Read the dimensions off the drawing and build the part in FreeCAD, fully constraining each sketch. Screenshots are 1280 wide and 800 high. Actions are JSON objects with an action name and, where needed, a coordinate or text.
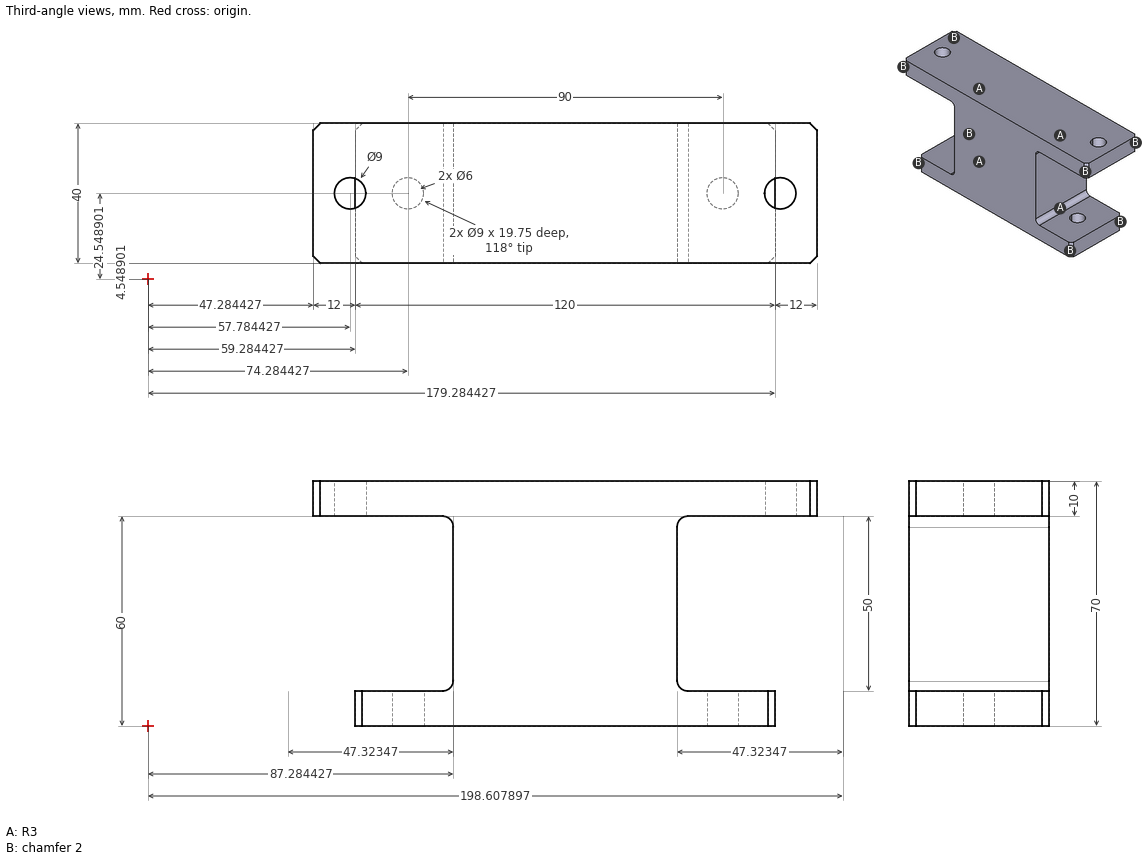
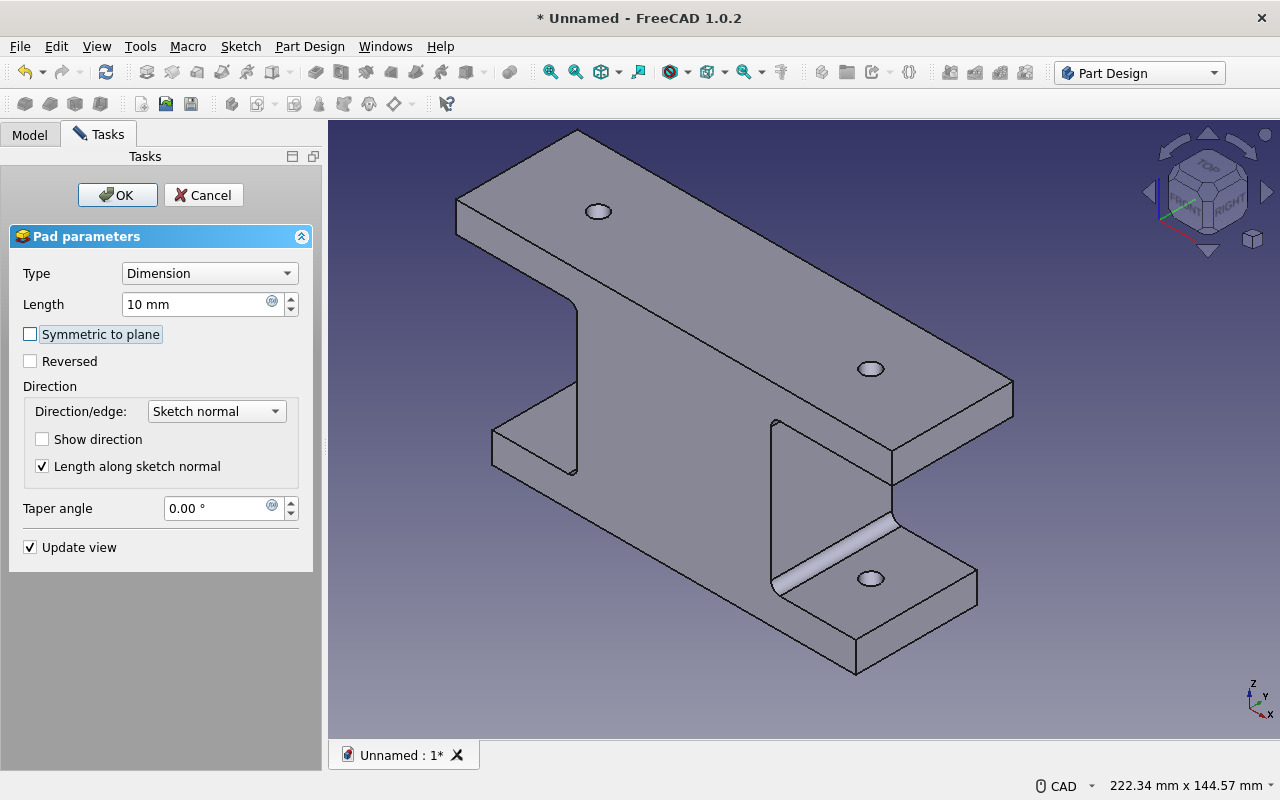
{"action": "left_click", "coordinate": [31, 361]}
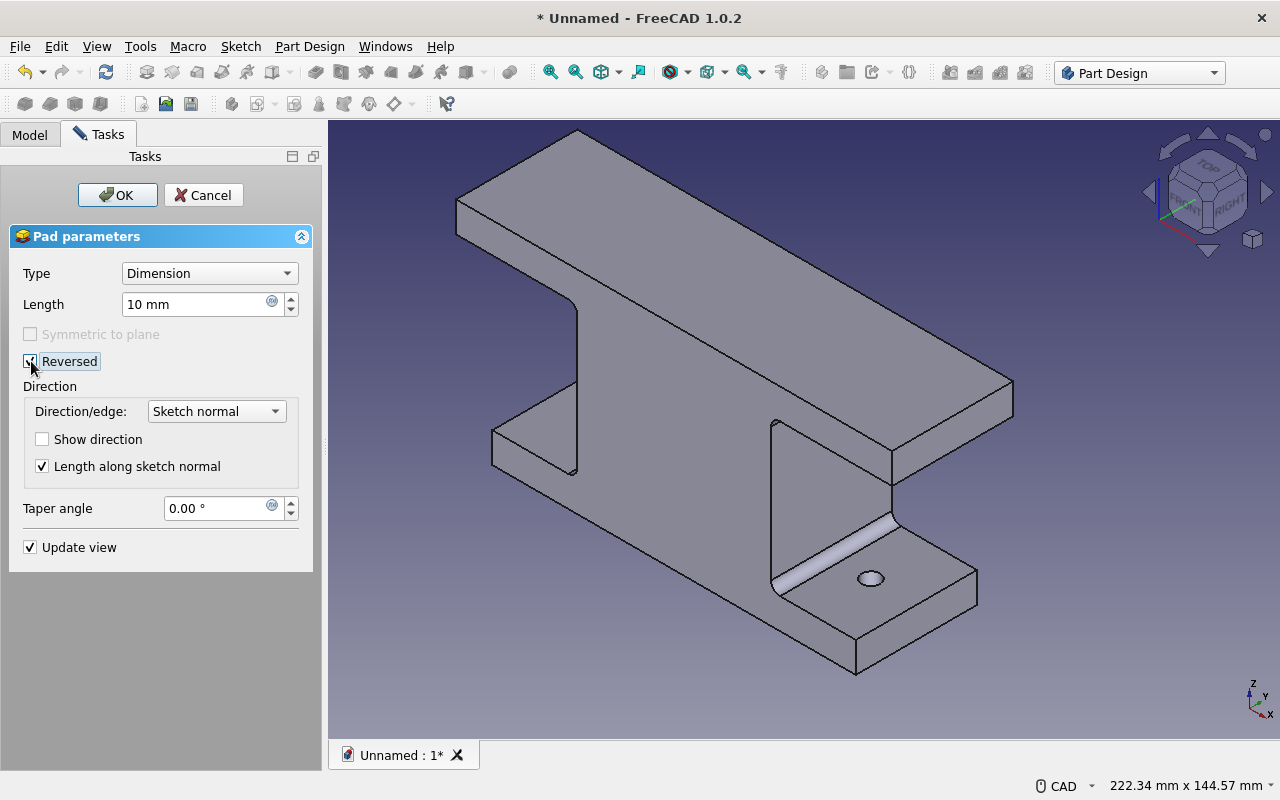
{"action": "left_click", "coordinate": [118, 195]}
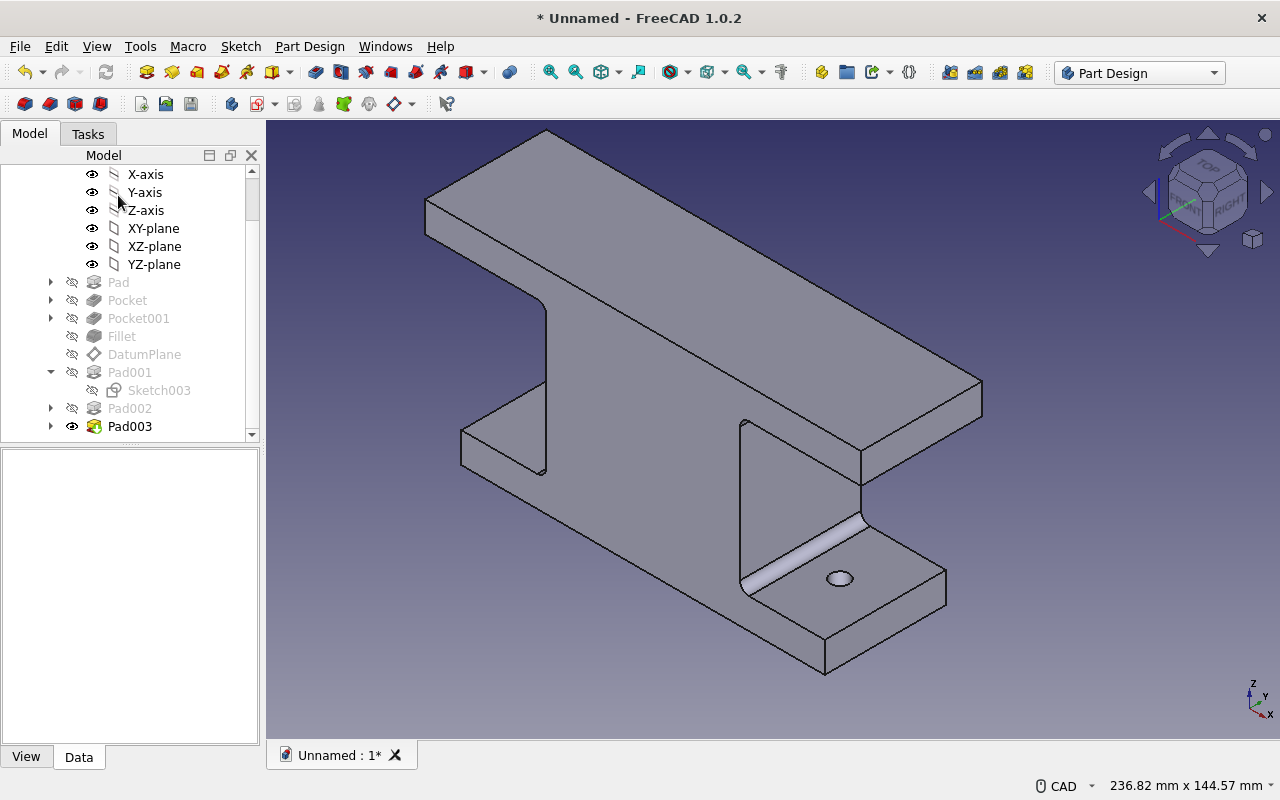
{"action": "left_click", "coordinate": [828, 361]}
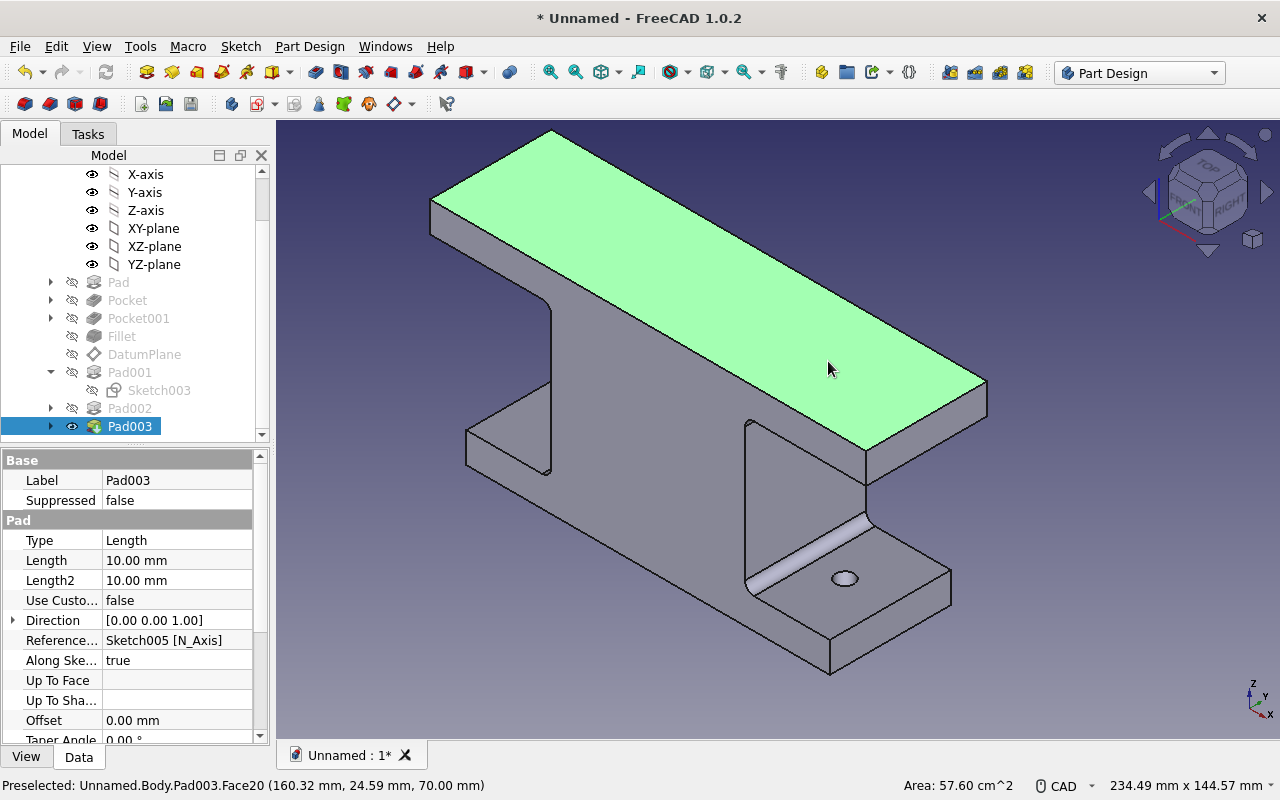
{"action": "left_click", "coordinate": [256, 104]}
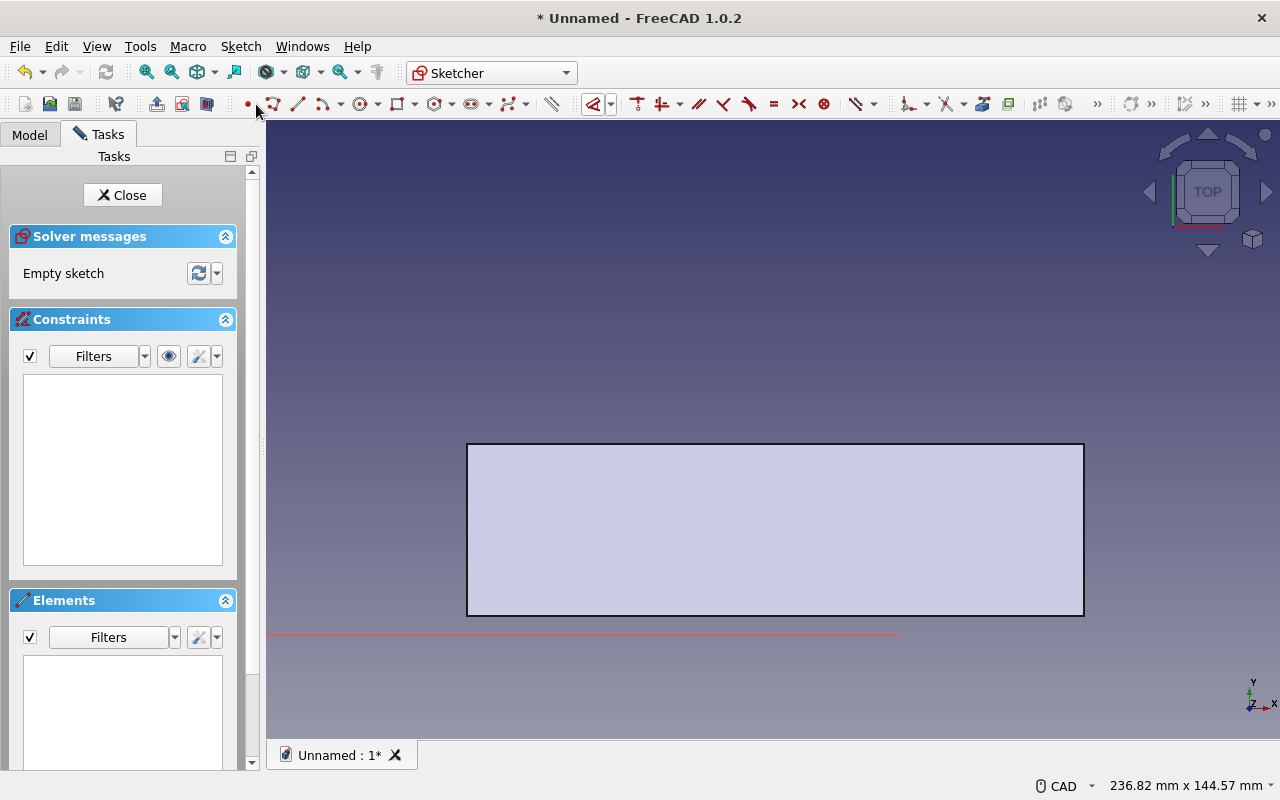
{"action": "scroll", "coordinate": [493, 540], "scroll_direction": "up", "scroll_amount": 12}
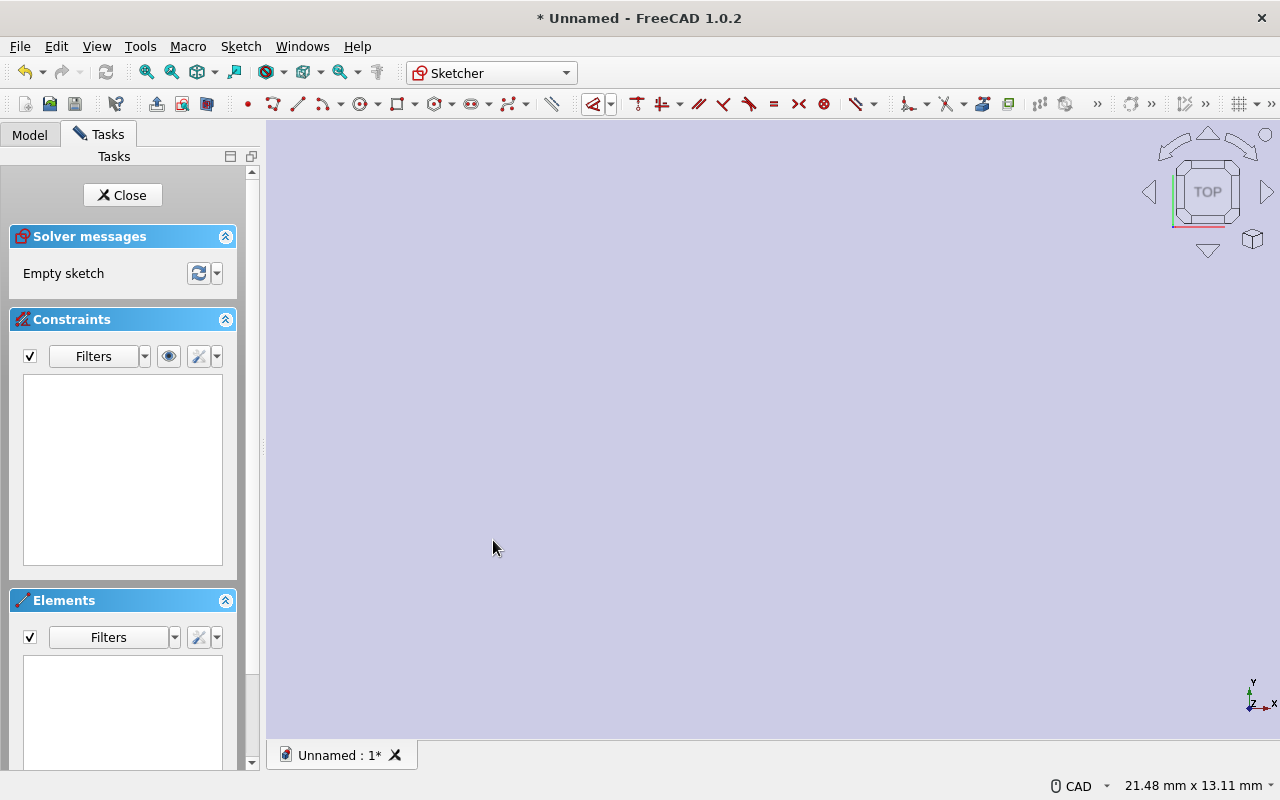
{"action": "left_click", "coordinate": [360, 104]}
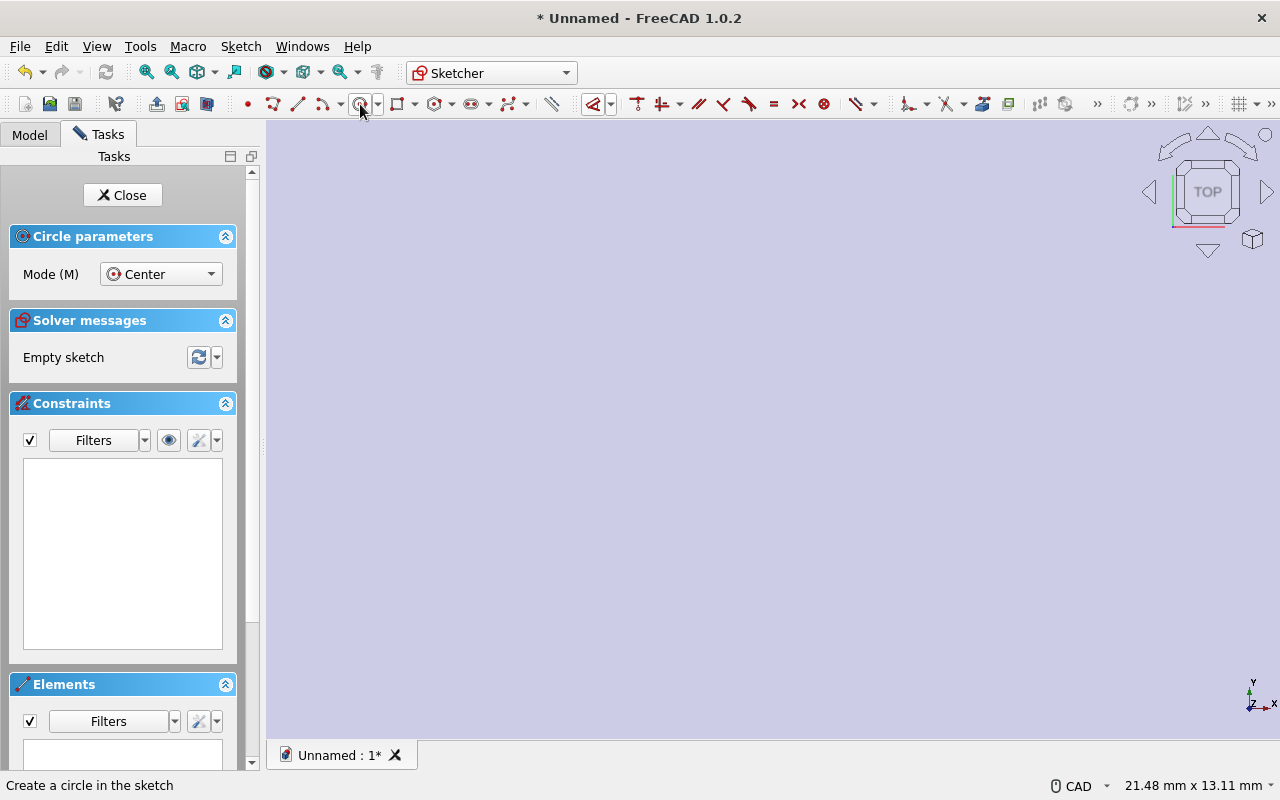
{"action": "left_click", "coordinate": [701, 422]}
{"action": "left_click", "coordinate": [851, 272]}
{"action": "key", "text": "Escape"}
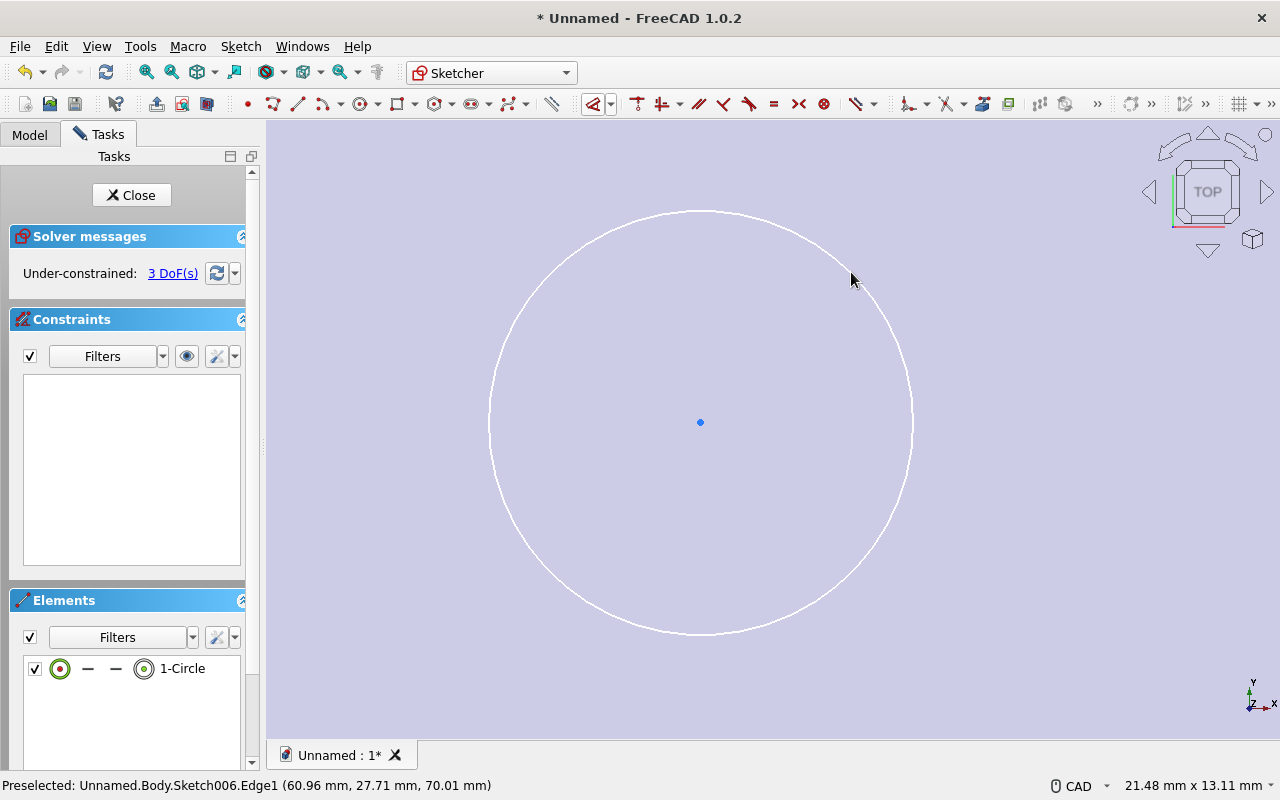
{"action": "left_click", "coordinate": [851, 273]}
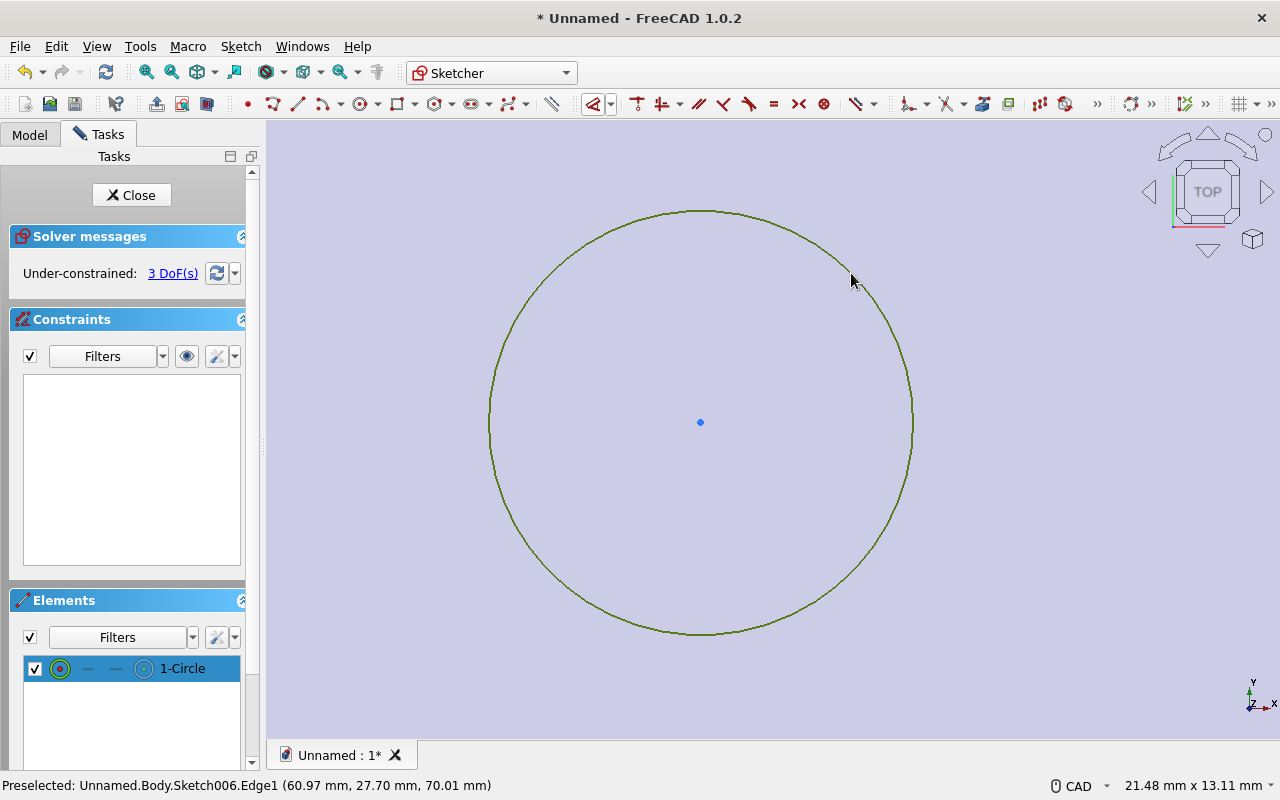
{"action": "key", "text": "k o"}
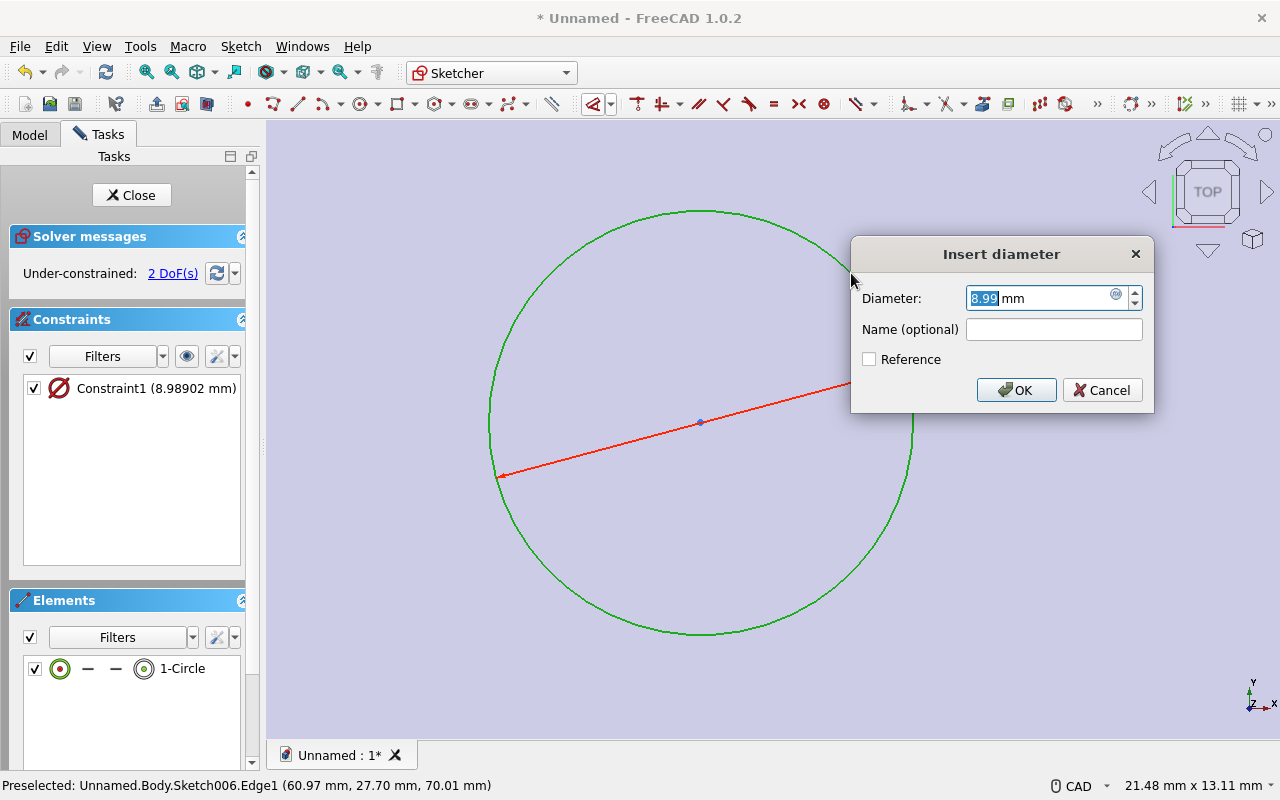
{"action": "type", "text": "9"}
{"action": "key", "text": "Return"}